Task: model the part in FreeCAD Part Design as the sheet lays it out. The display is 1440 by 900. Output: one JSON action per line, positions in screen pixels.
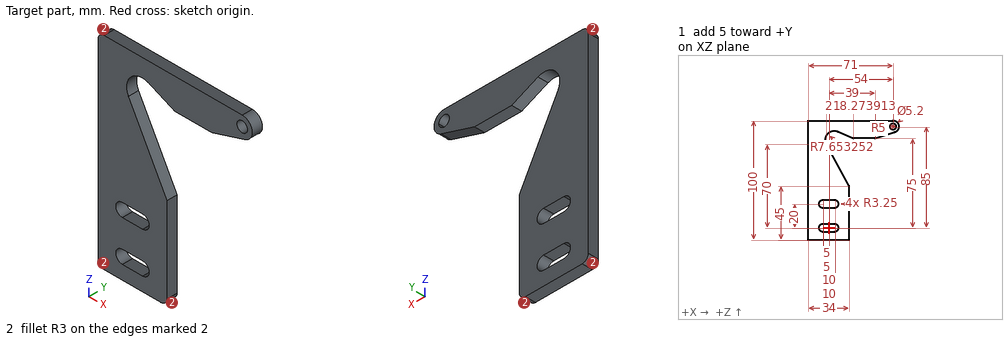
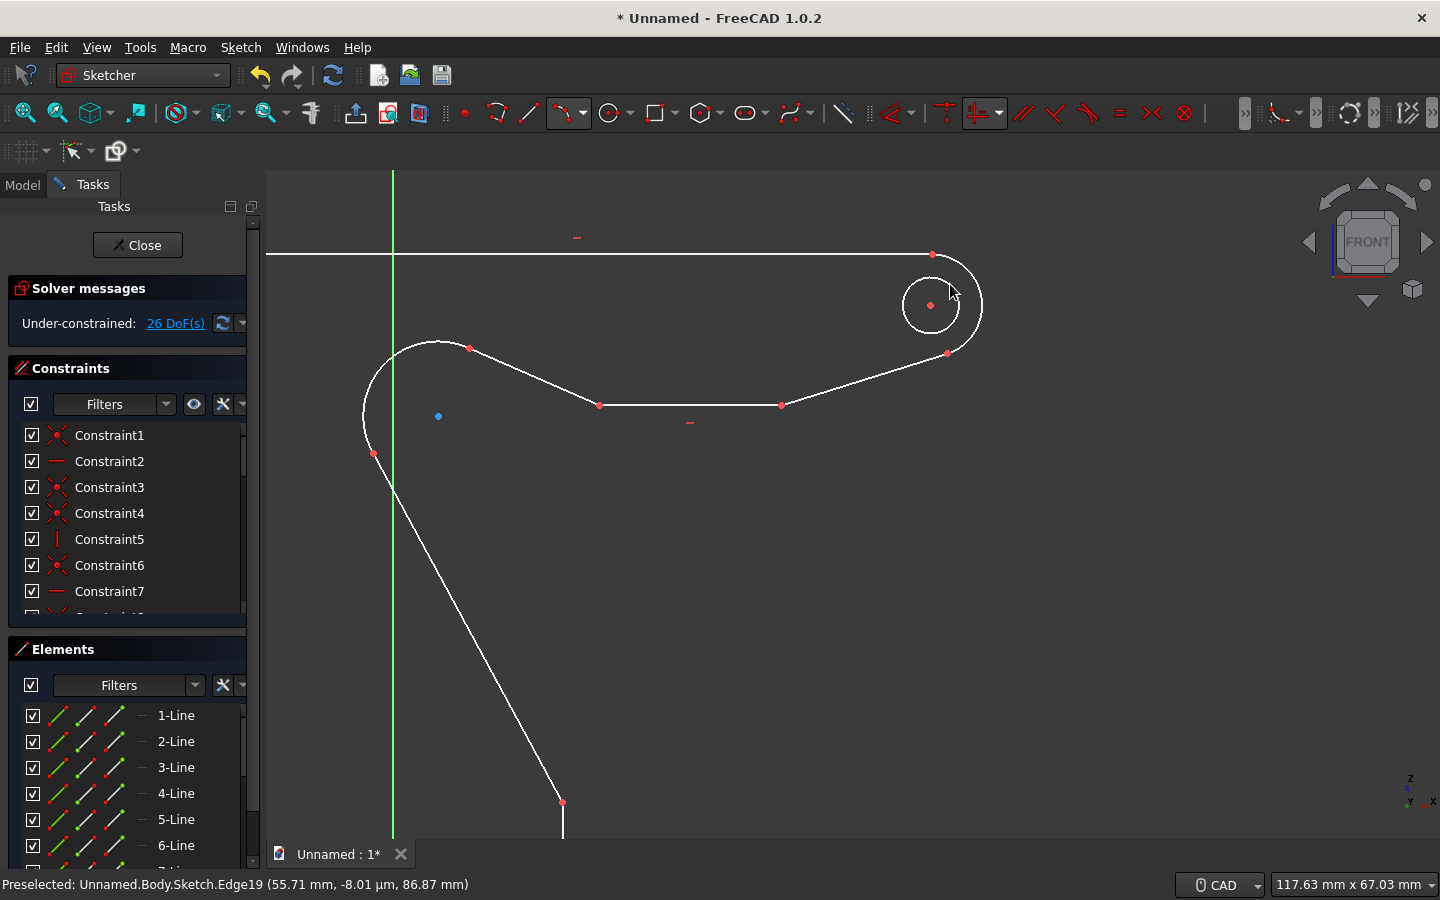
{"action": "left_click", "coordinate": [898, 369]}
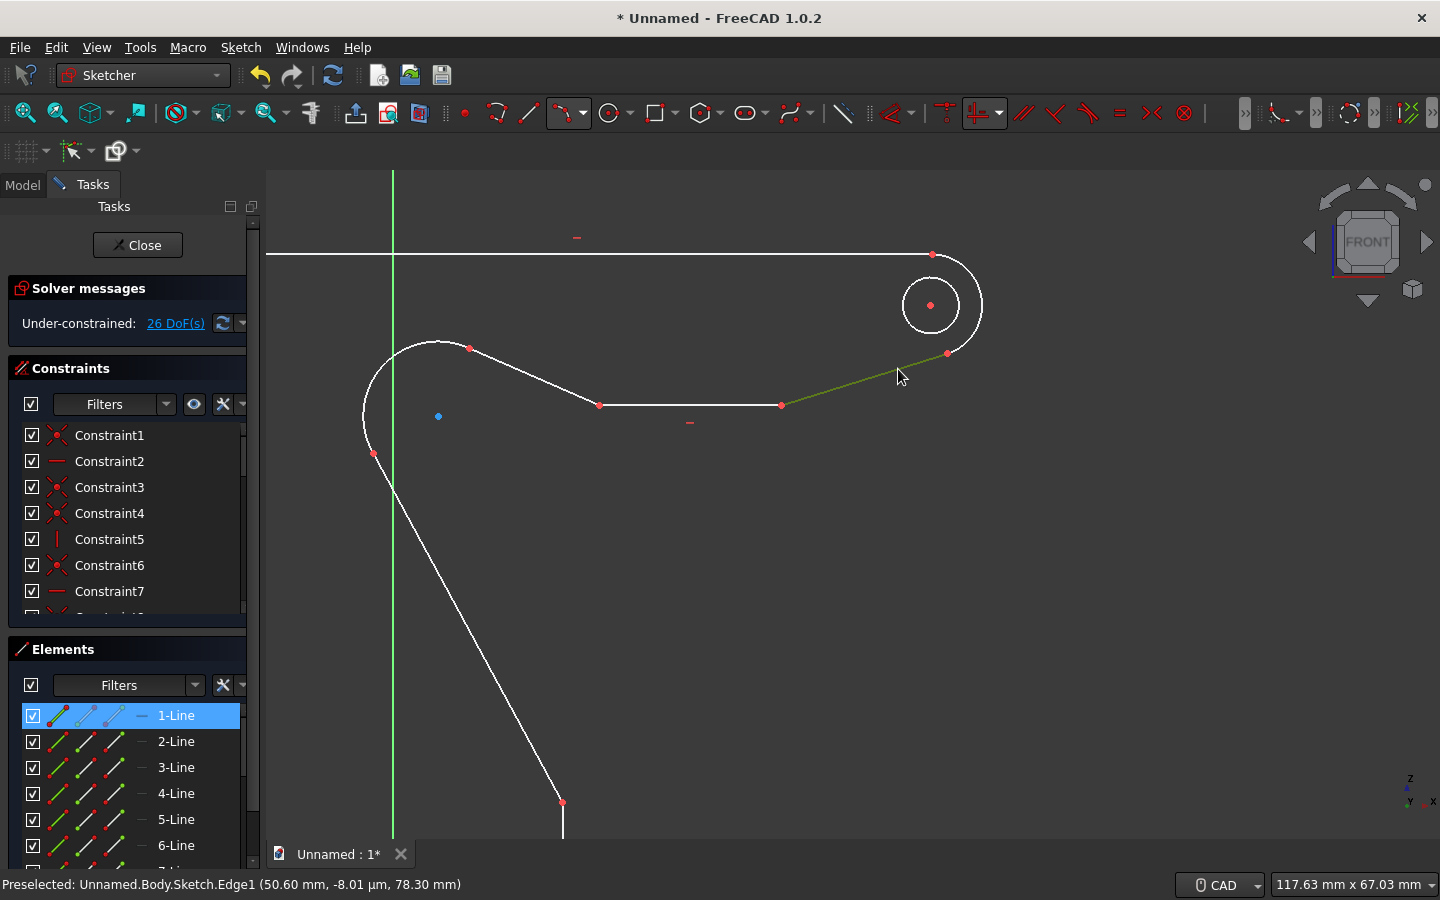
{"action": "left_click", "coordinate": [978, 326]}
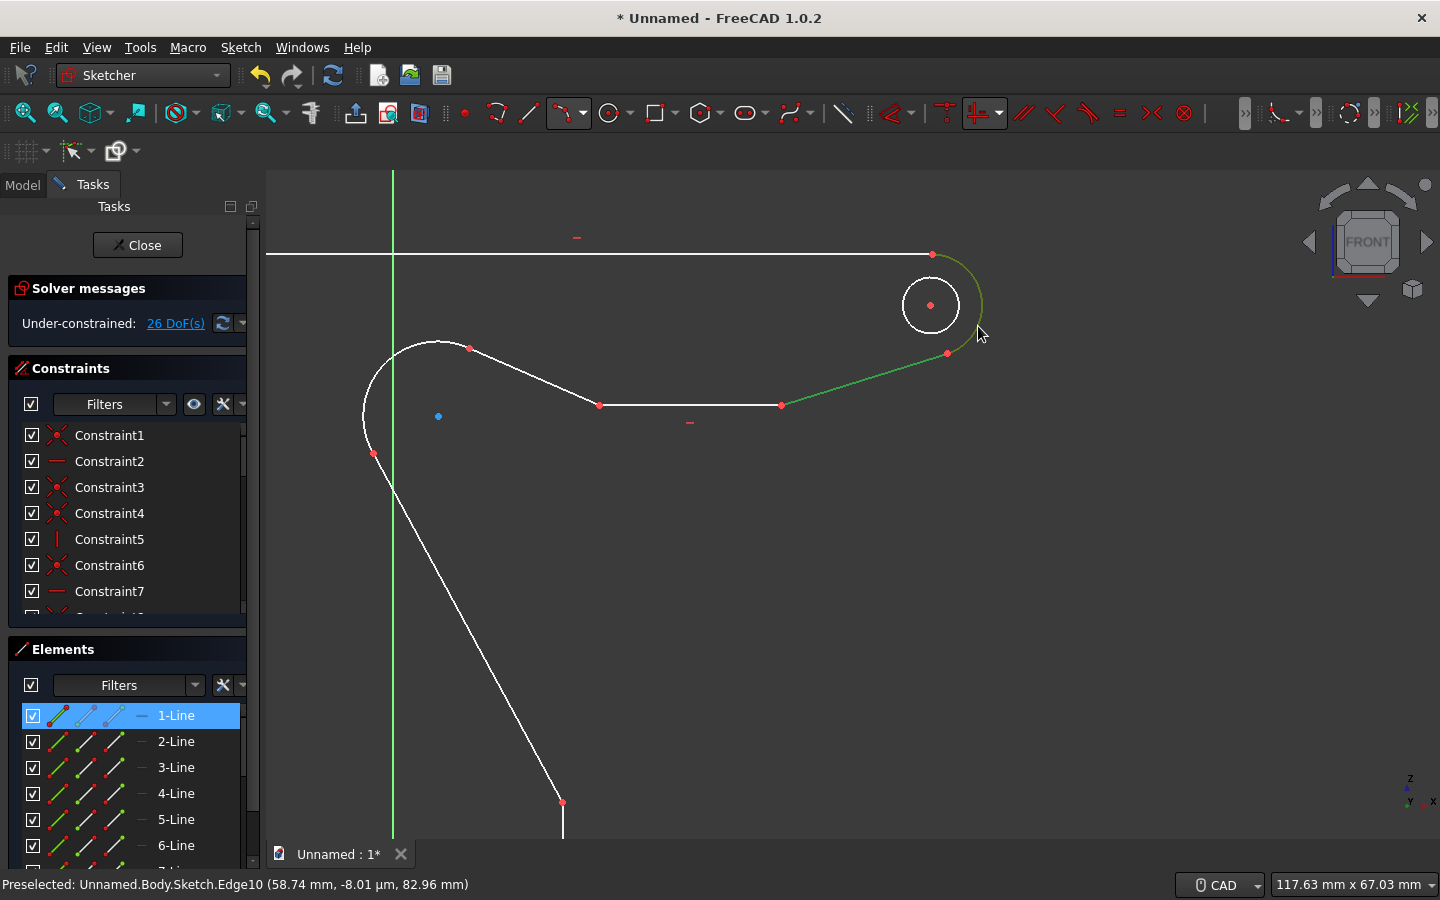
{"action": "key", "text": "t"}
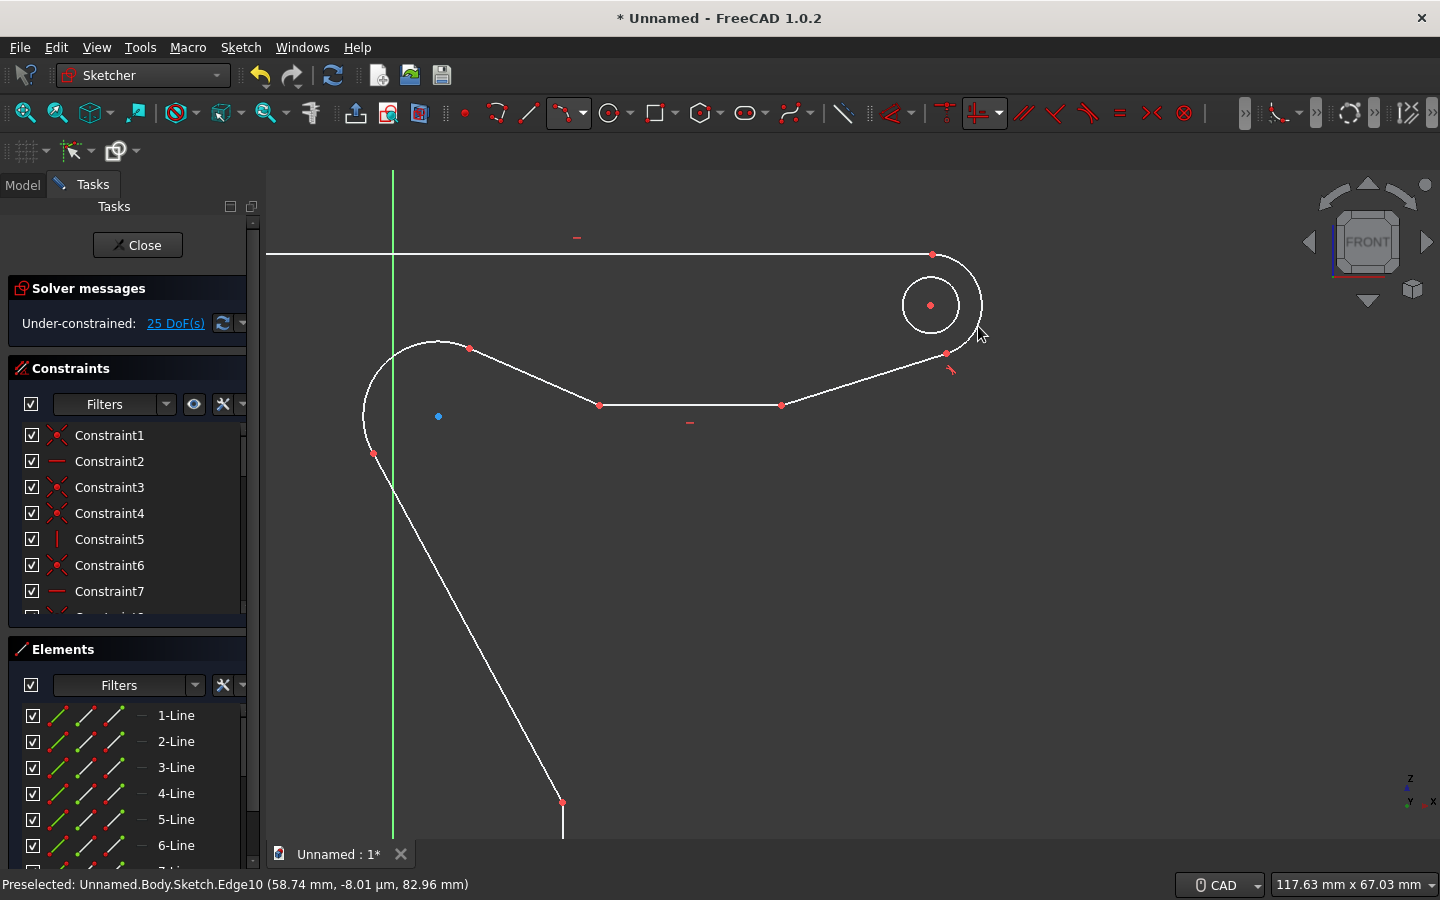
{"action": "left_click", "coordinate": [561, 388]}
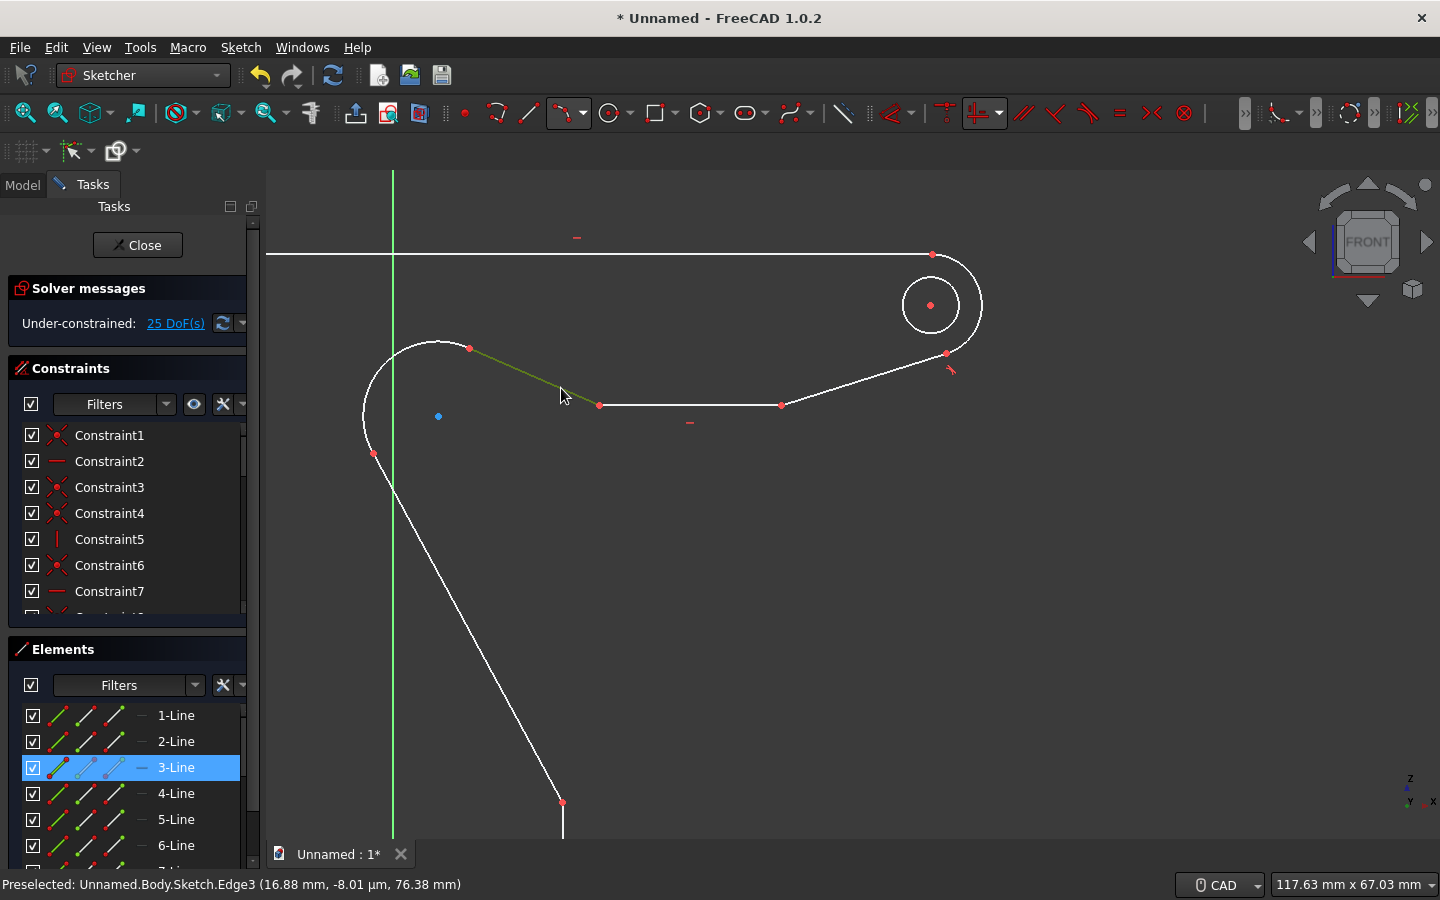
{"action": "left_click", "coordinate": [414, 345]}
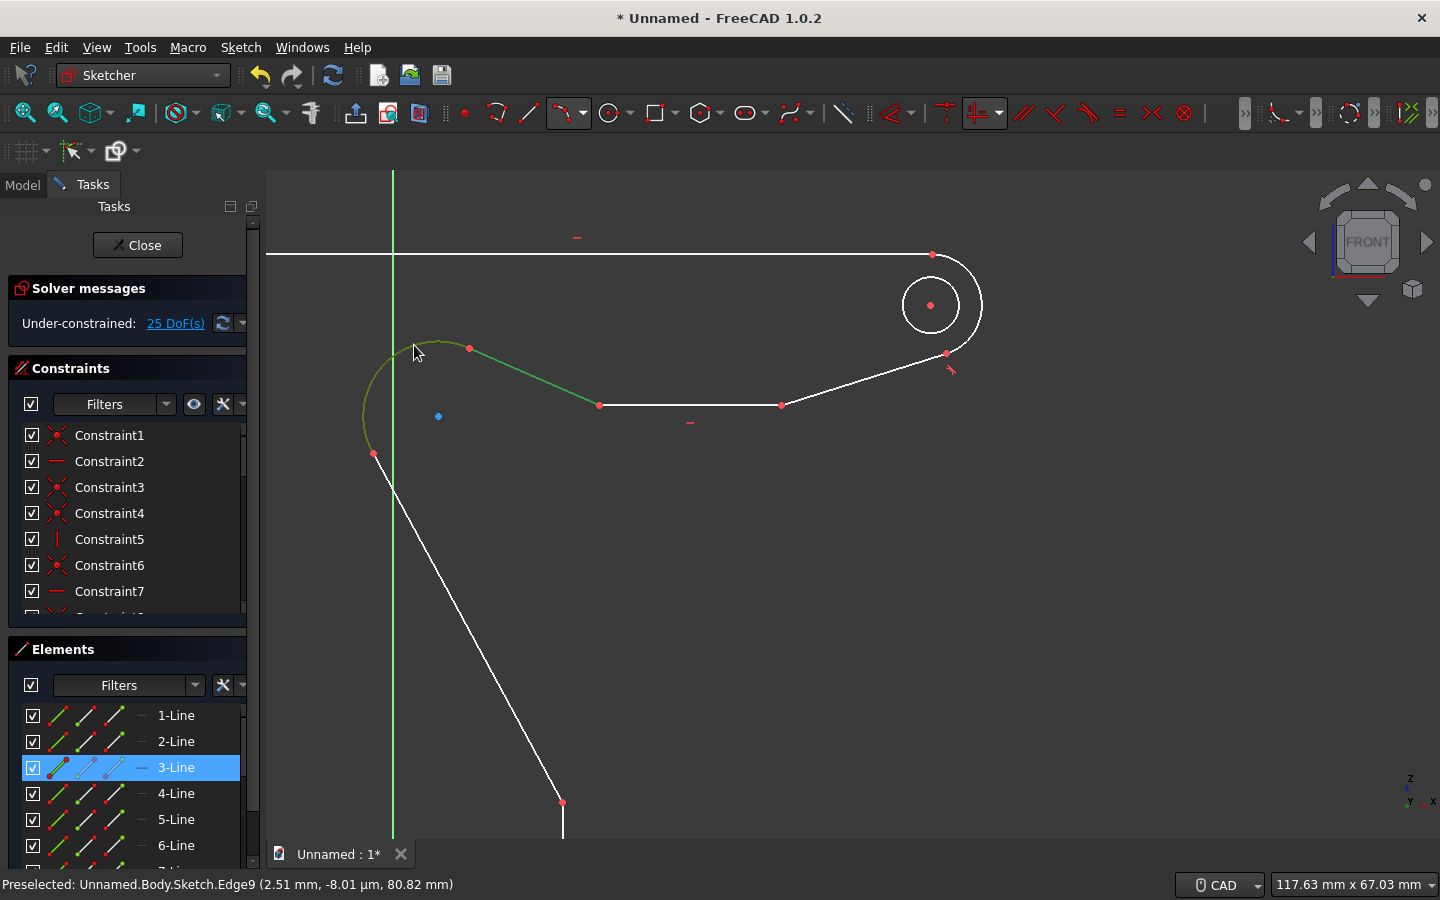
{"action": "left_click", "coordinate": [1088, 114]}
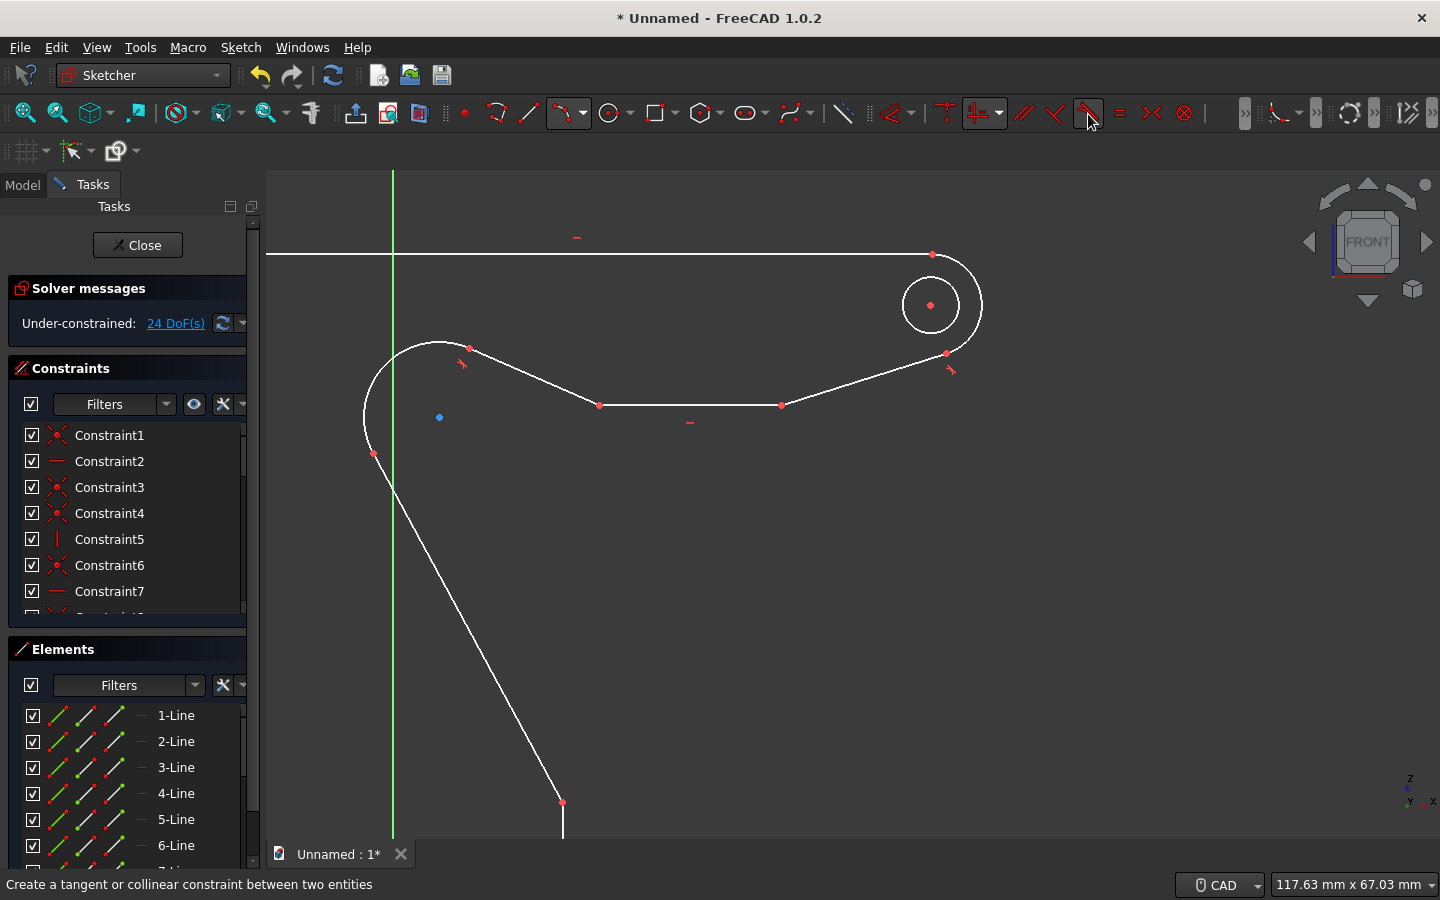
{"action": "left_click", "coordinate": [430, 558]}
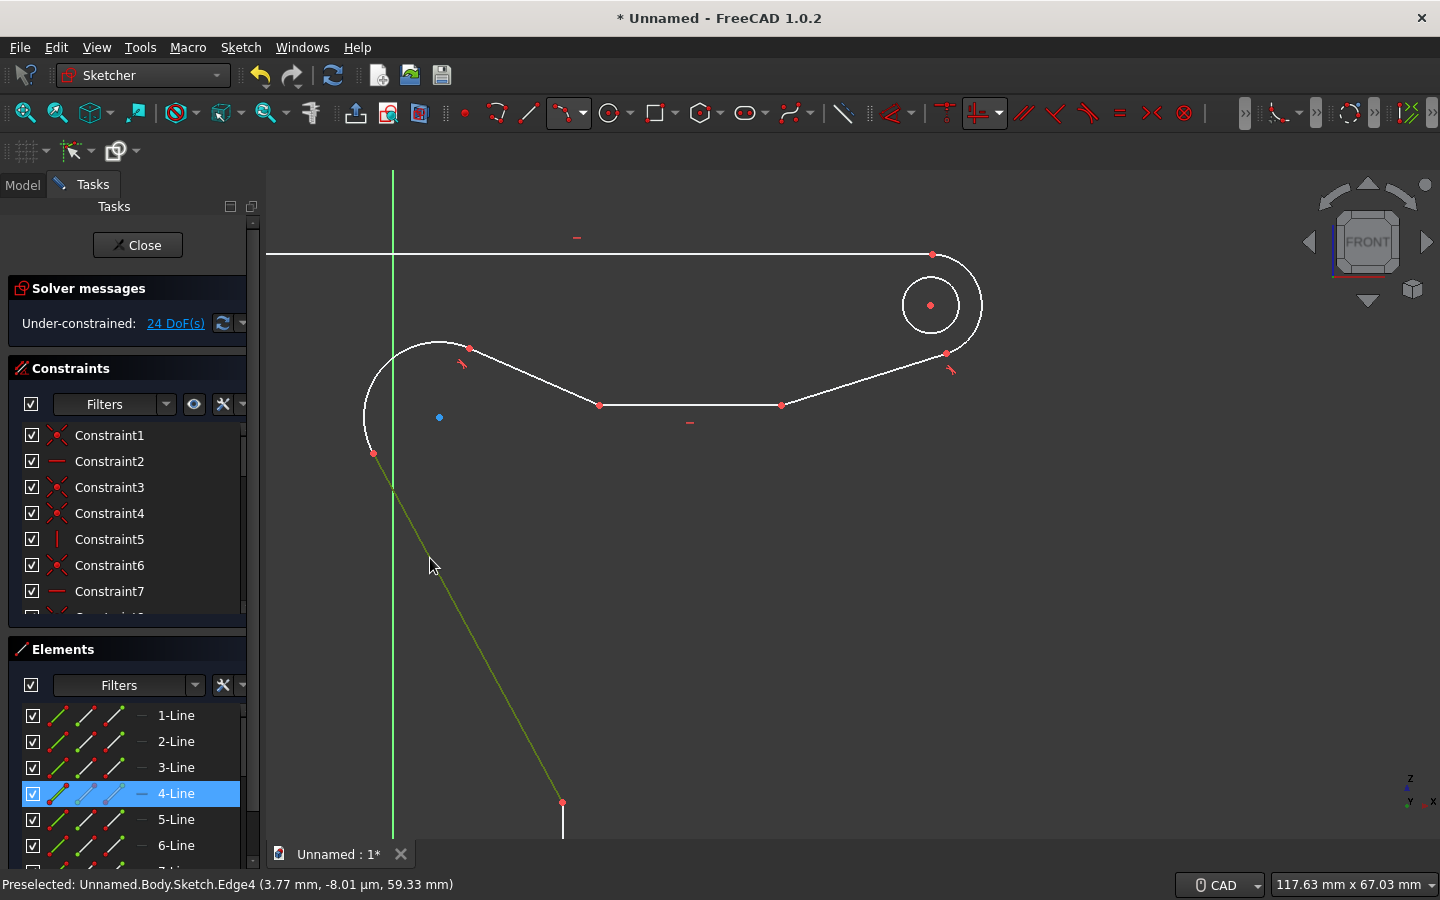
{"action": "left_click", "coordinate": [415, 346]}